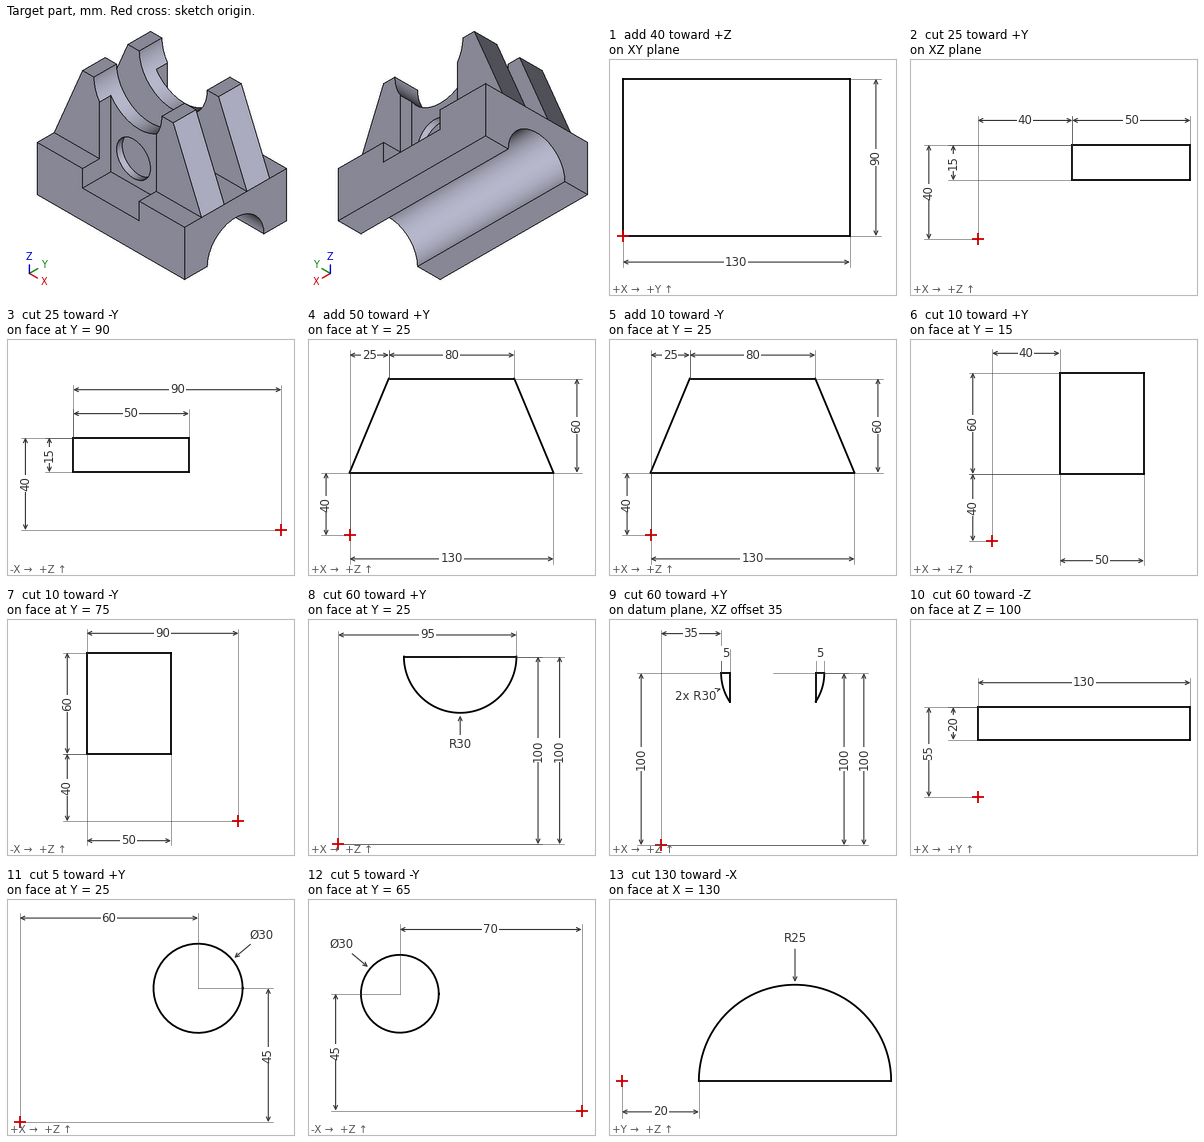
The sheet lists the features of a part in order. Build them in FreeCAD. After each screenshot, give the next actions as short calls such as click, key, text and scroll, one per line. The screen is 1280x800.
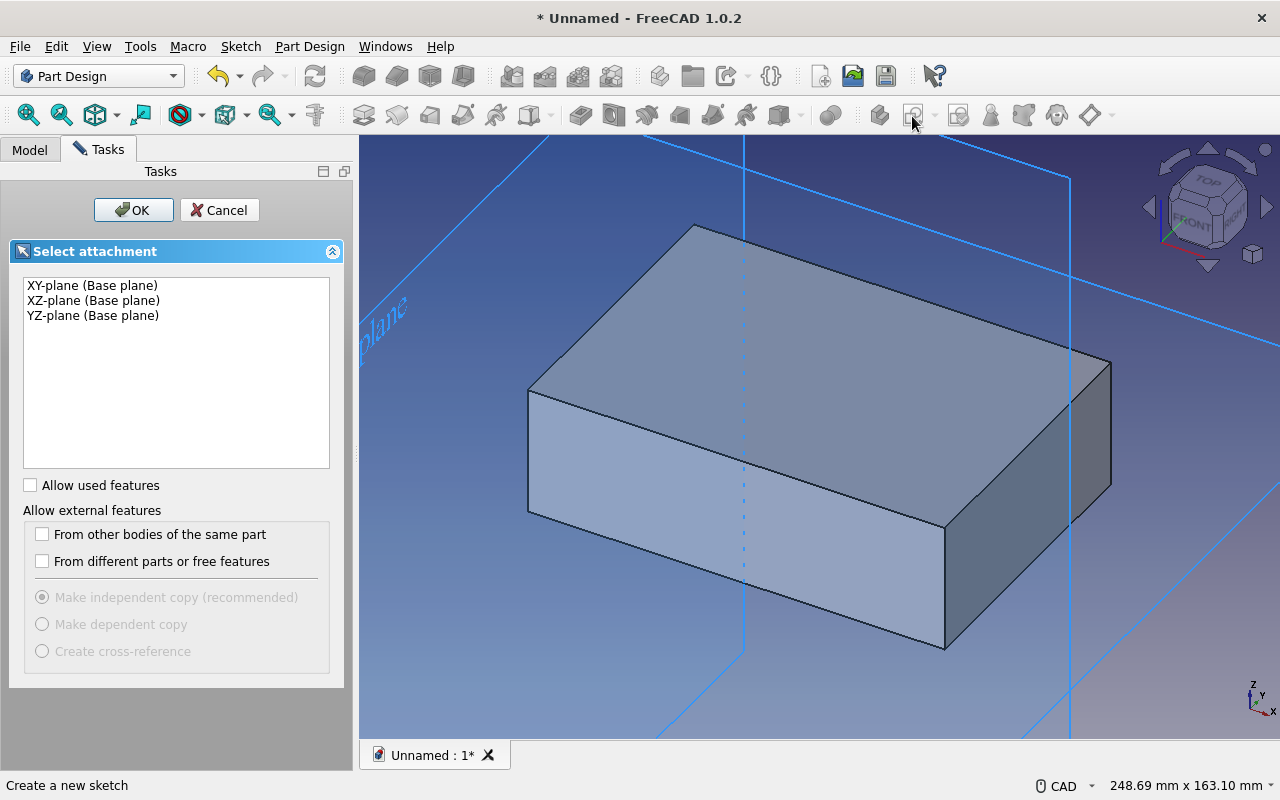
click(84, 300)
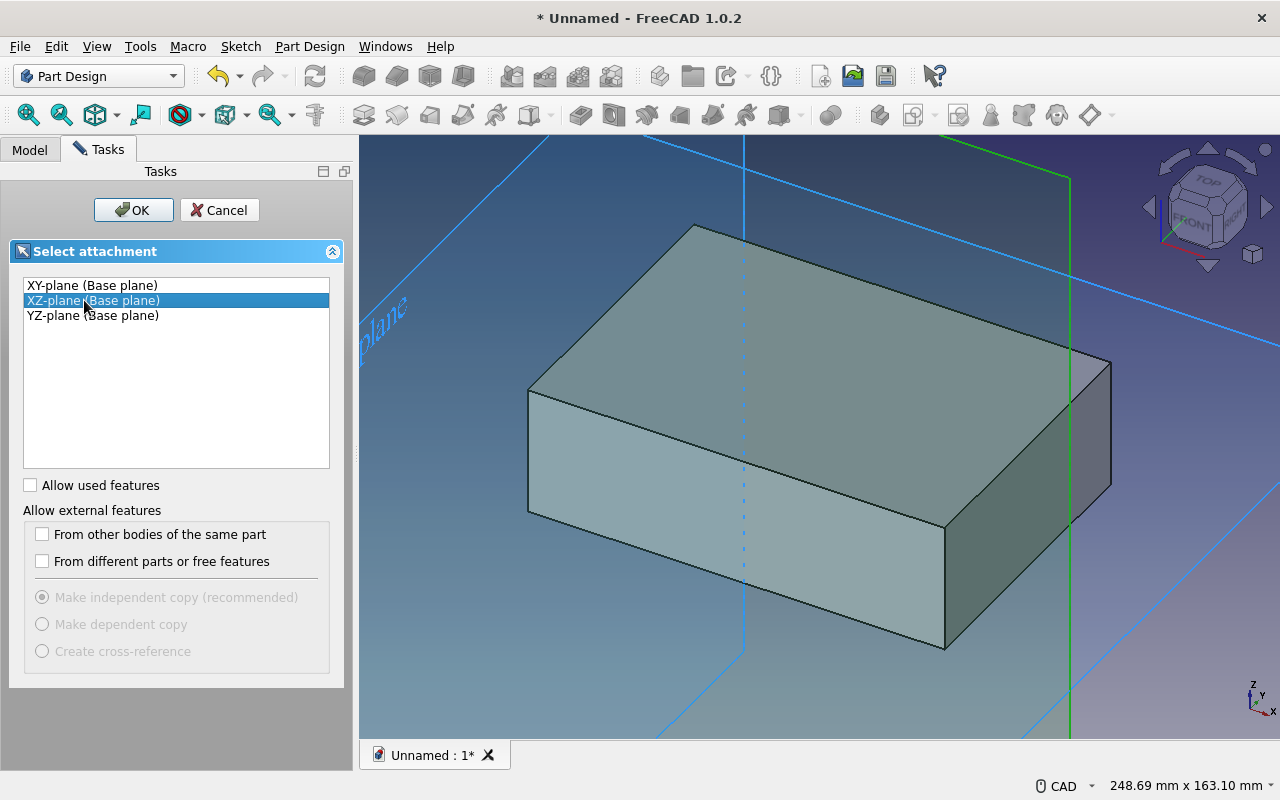
click(134, 210)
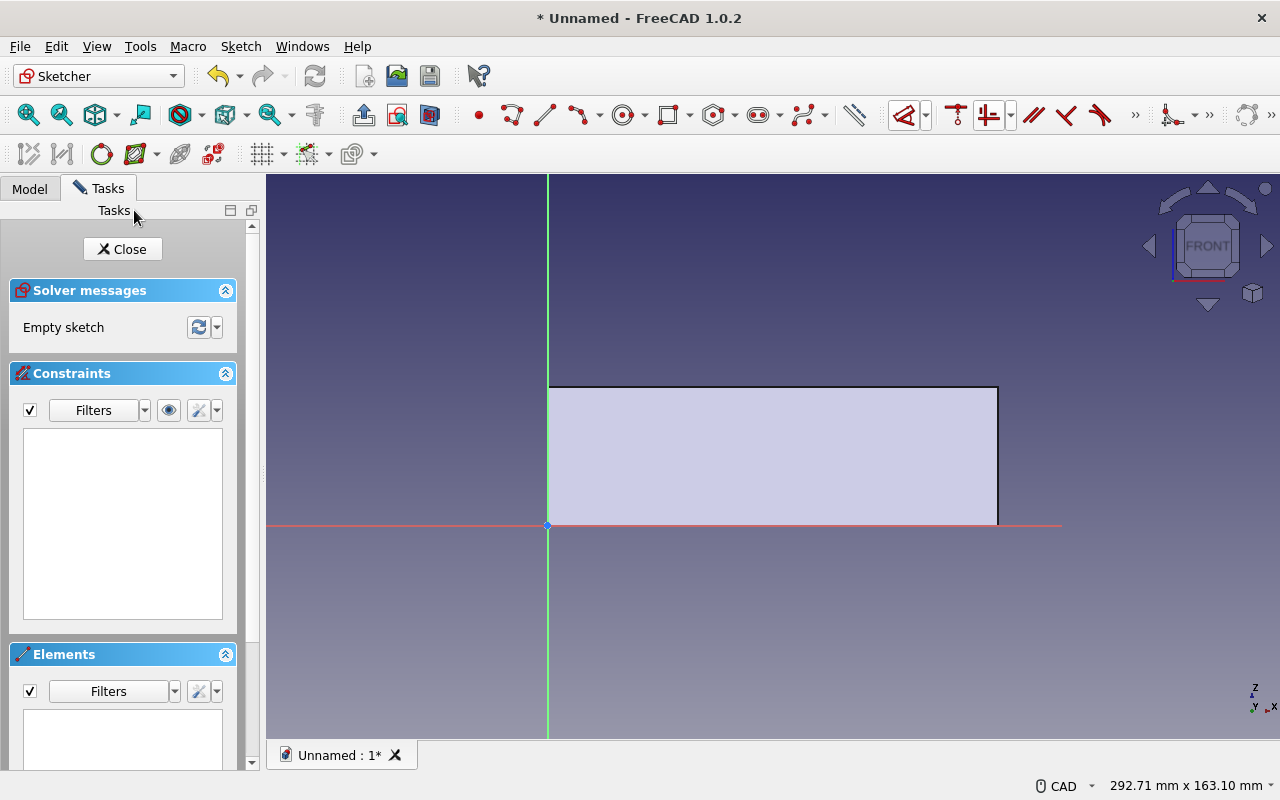
scroll(703, 456, up, 3)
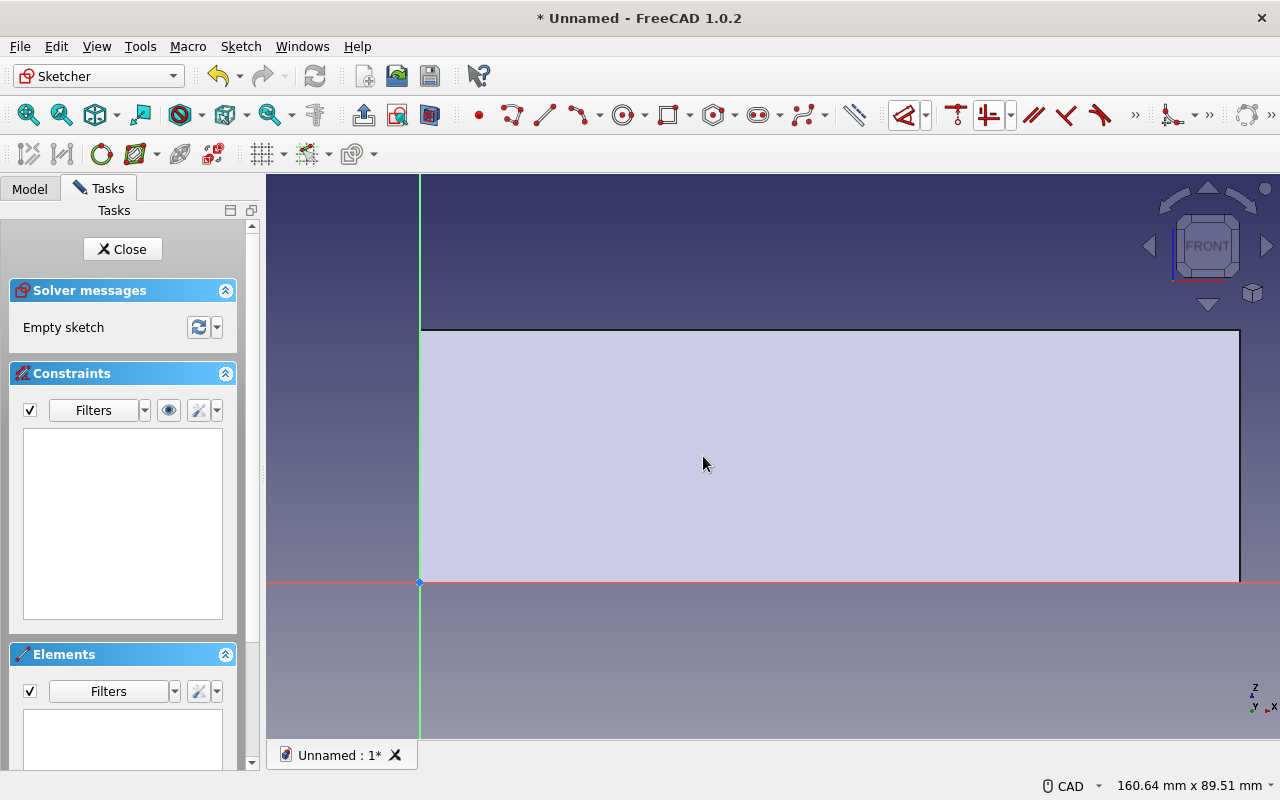
key(g)
key(r)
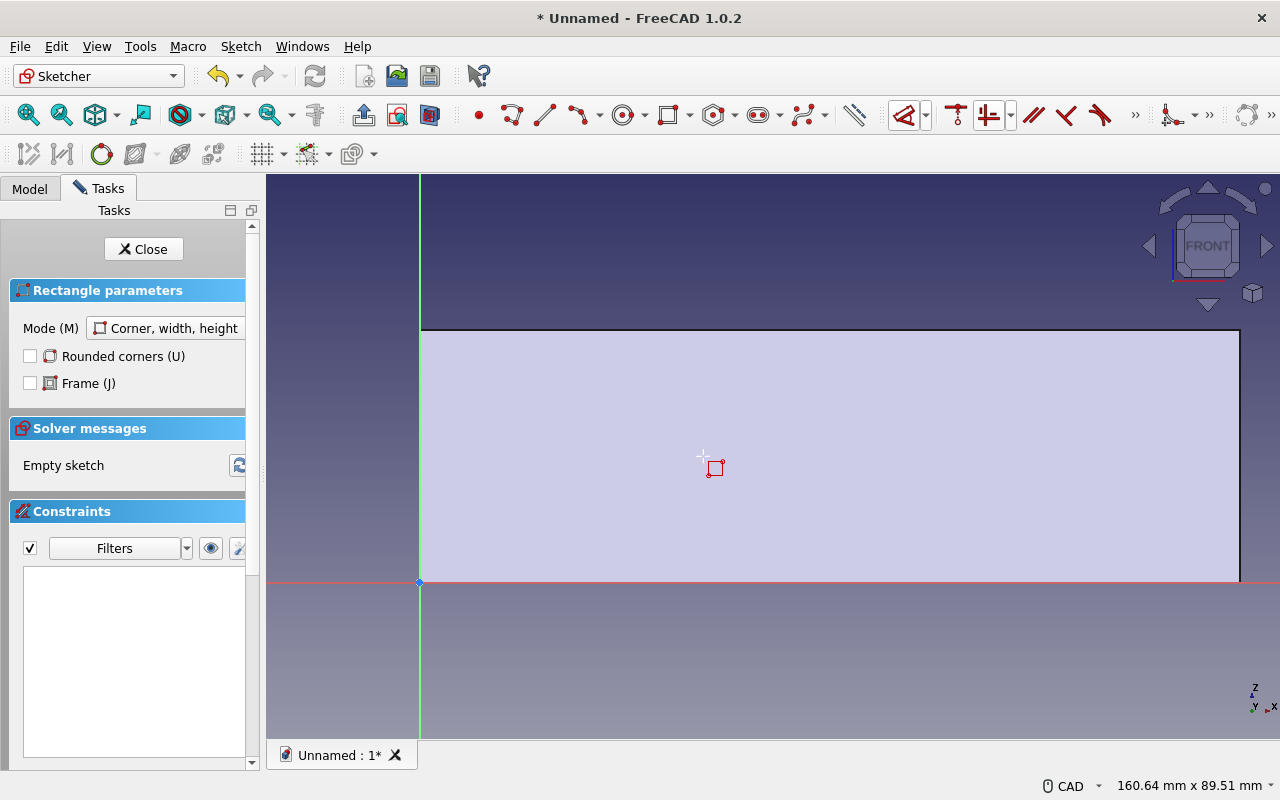
click(672, 330)
click(988, 425)
key(Escape)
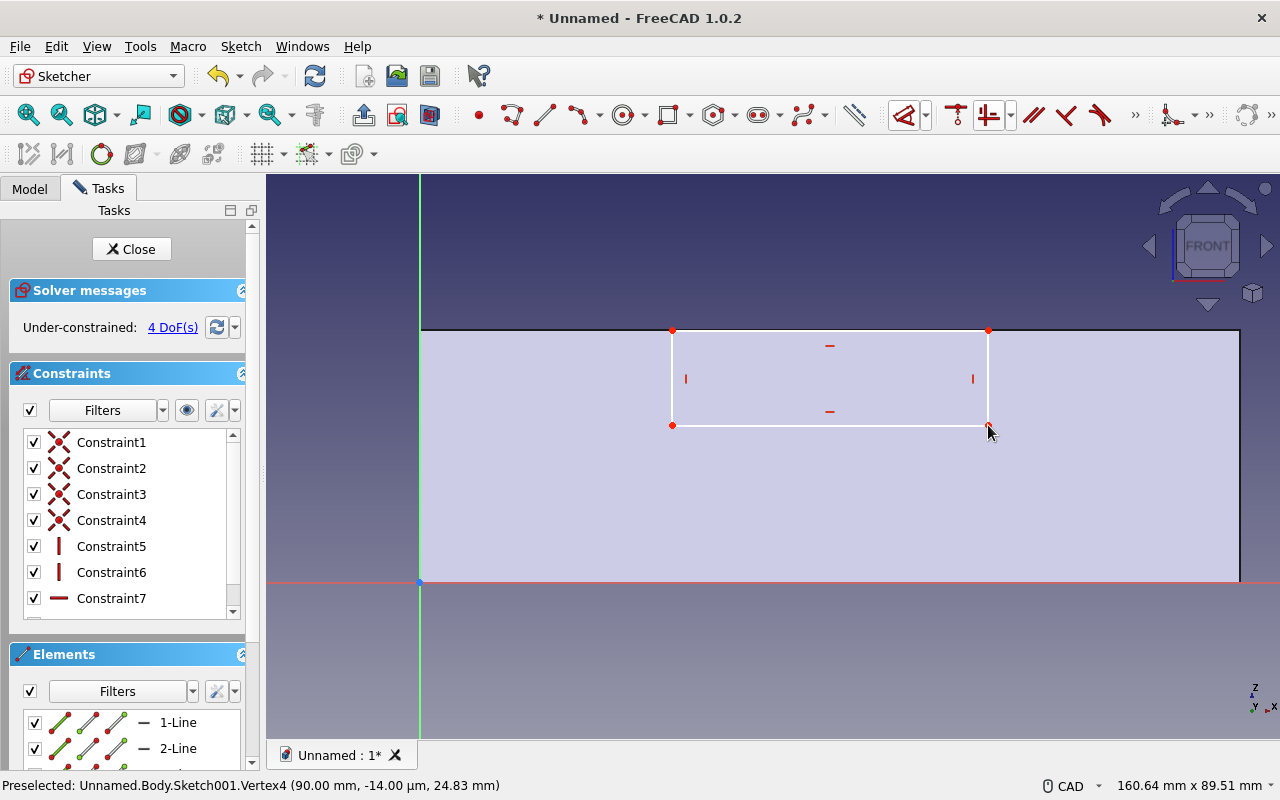
key(d)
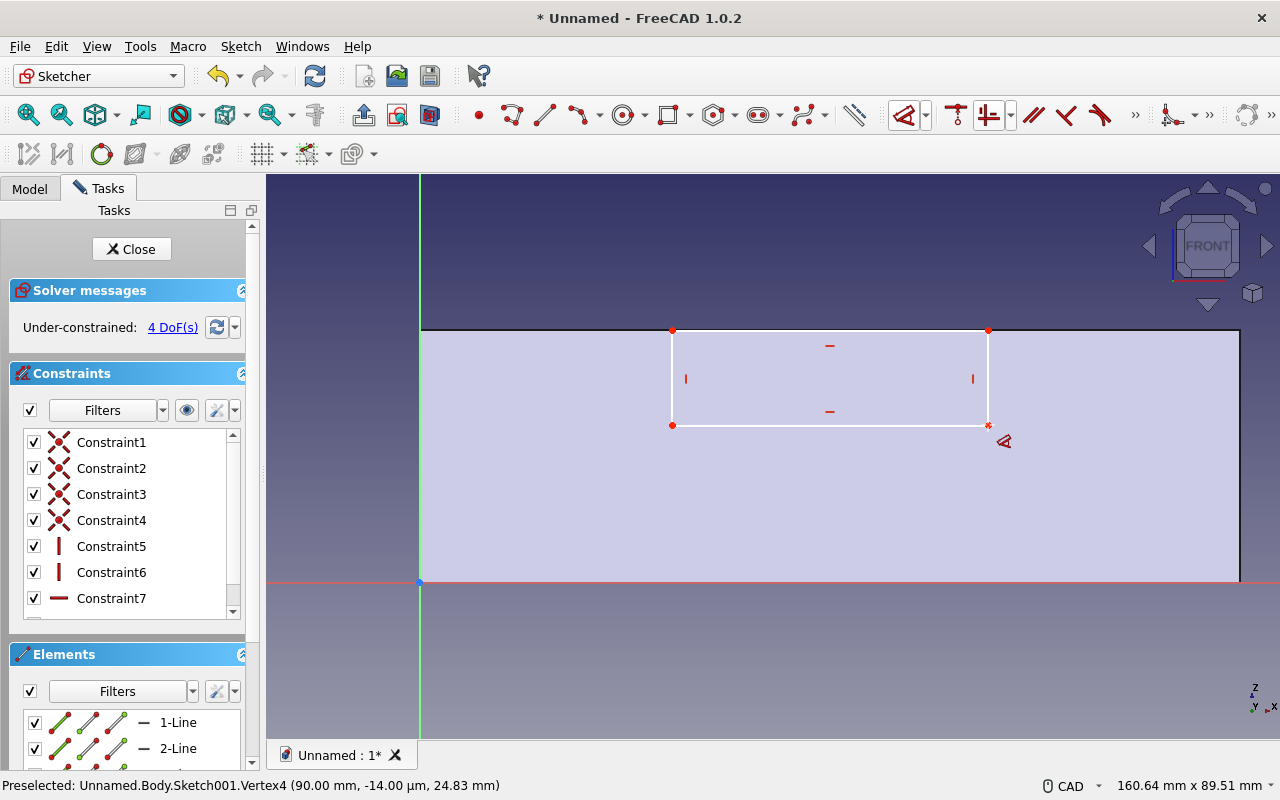
click(672, 359)
click(638, 378)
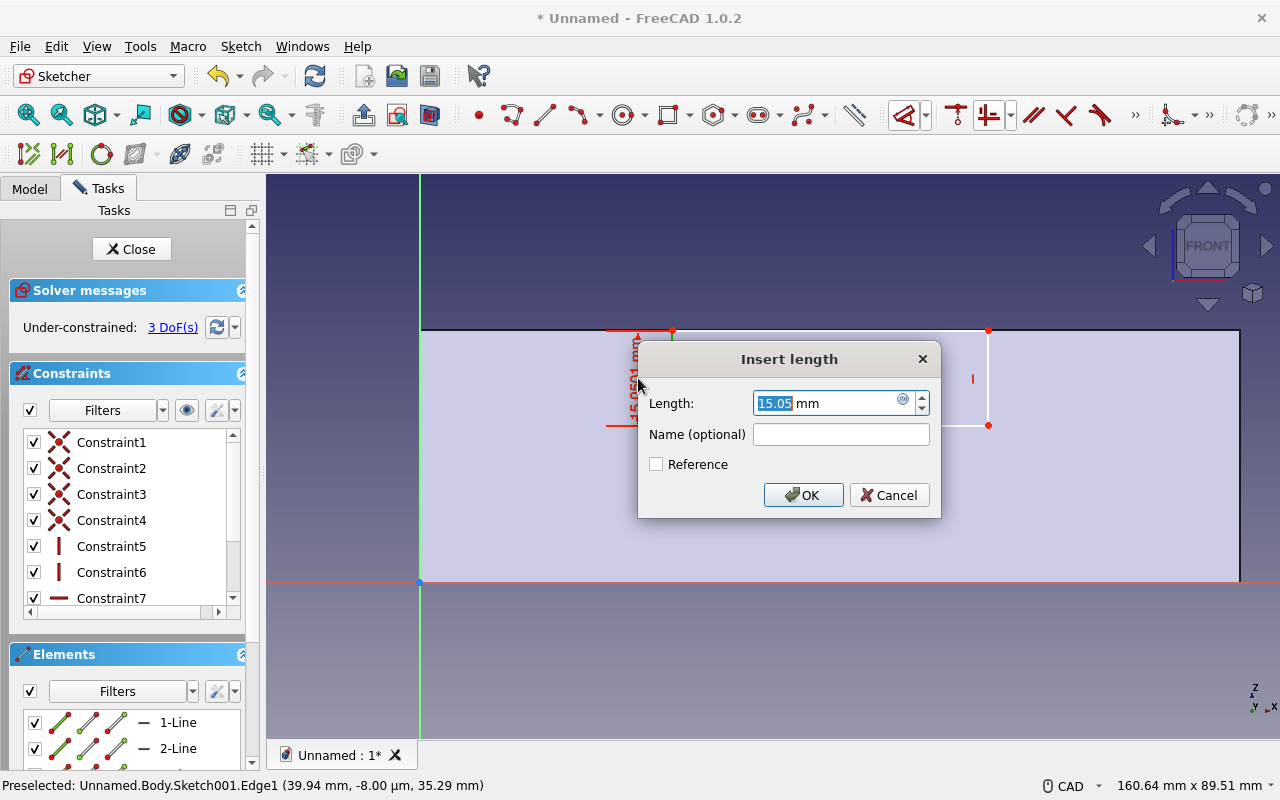
text(15)
key(Return)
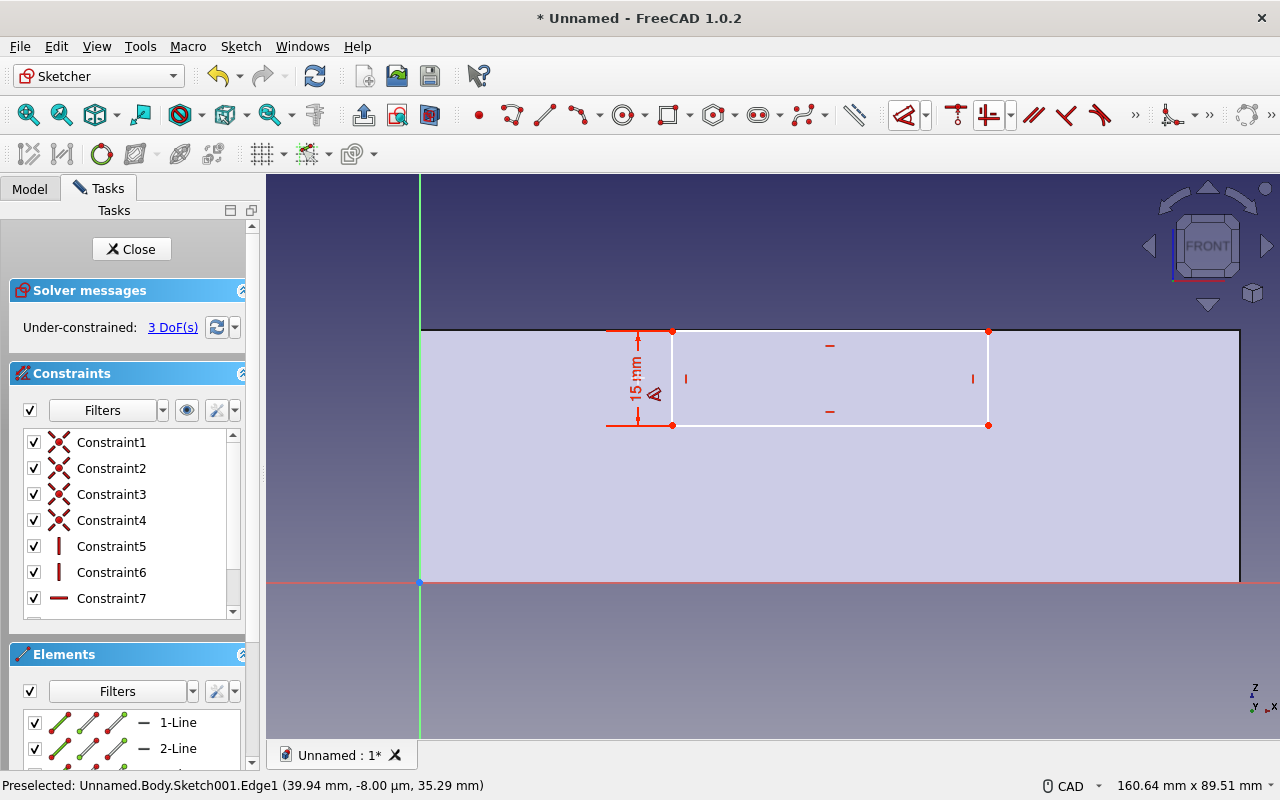
click(767, 426)
click(830, 392)